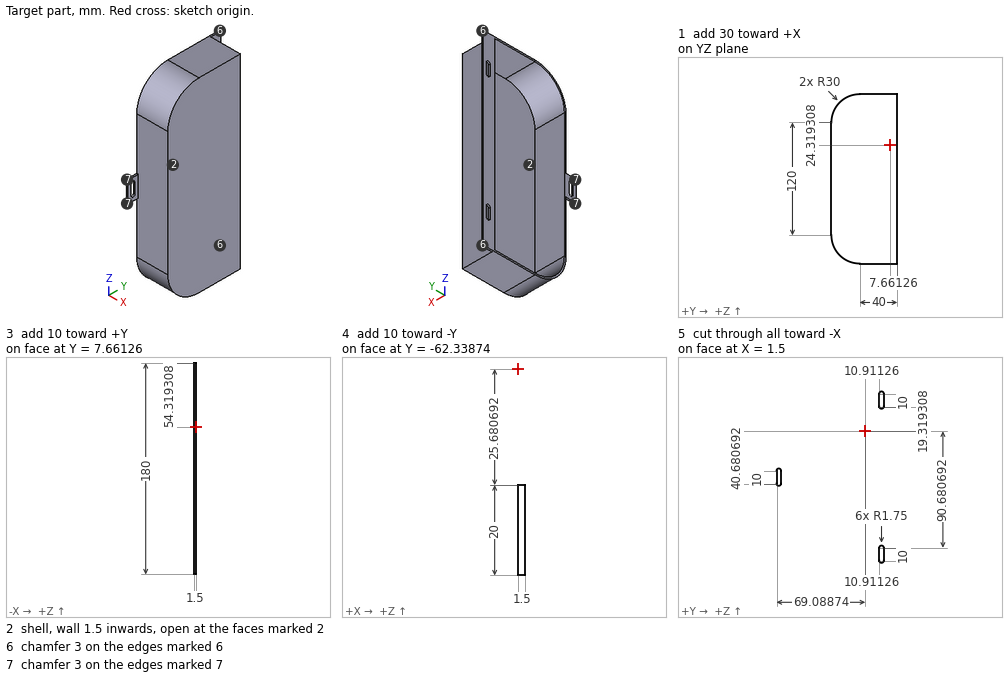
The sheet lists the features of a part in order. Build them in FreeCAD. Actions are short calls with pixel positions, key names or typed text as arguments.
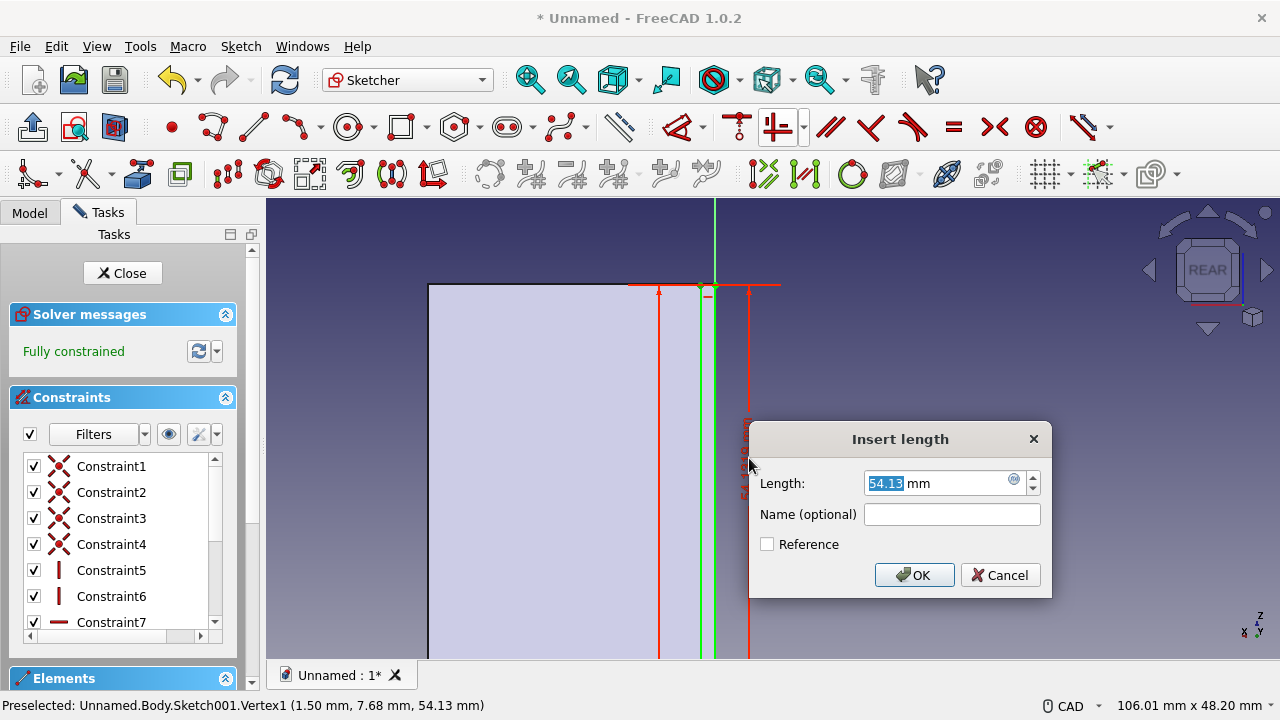
text(54.319308)
key(Return)
key(Escape)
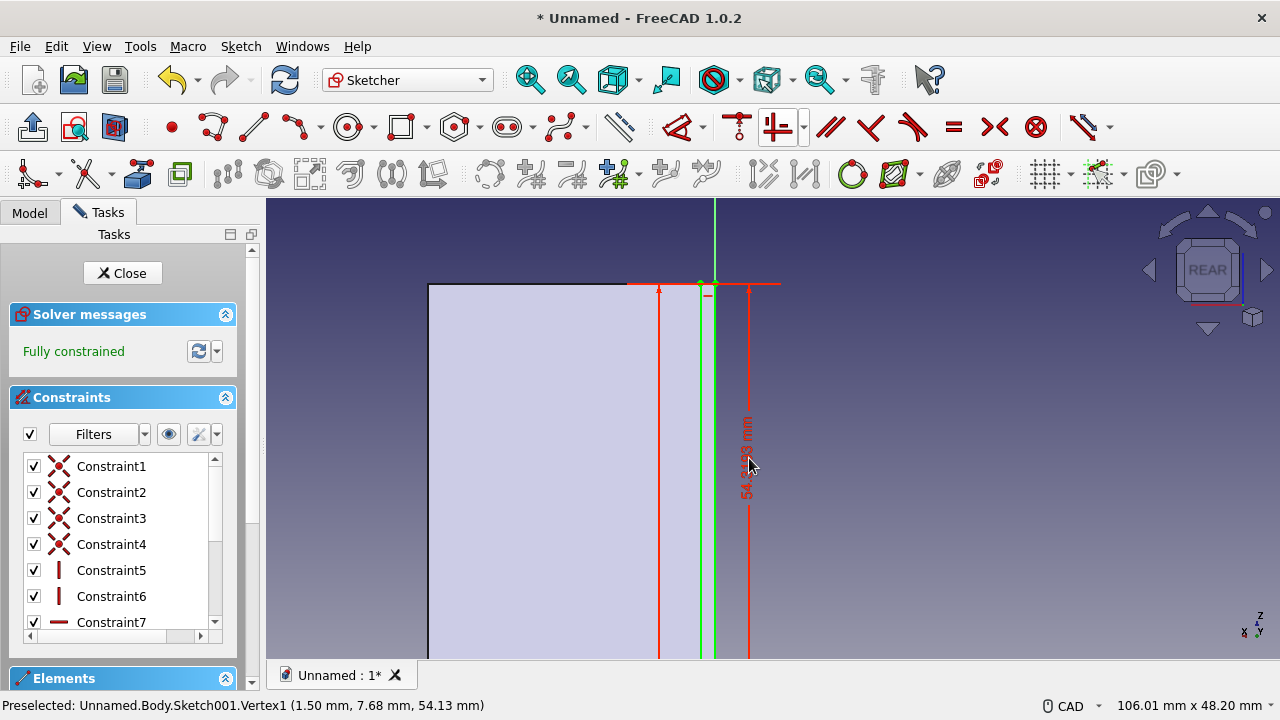
click(123, 273)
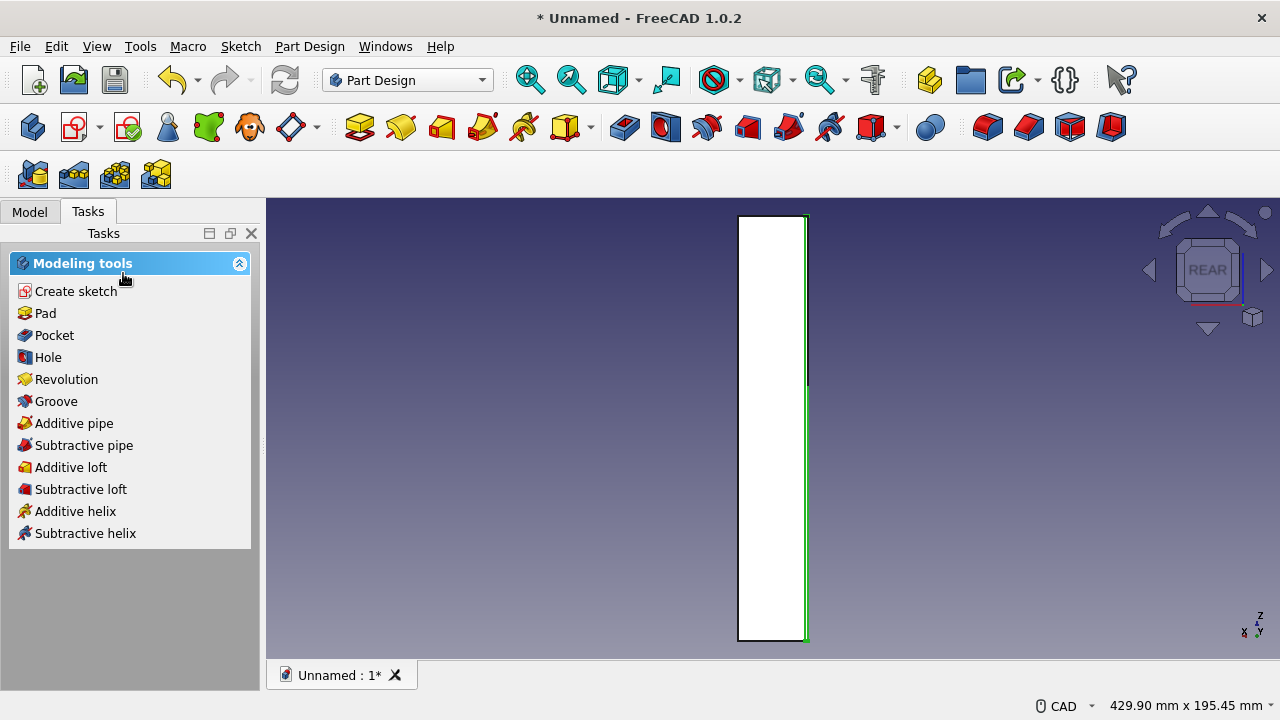
click(360, 128)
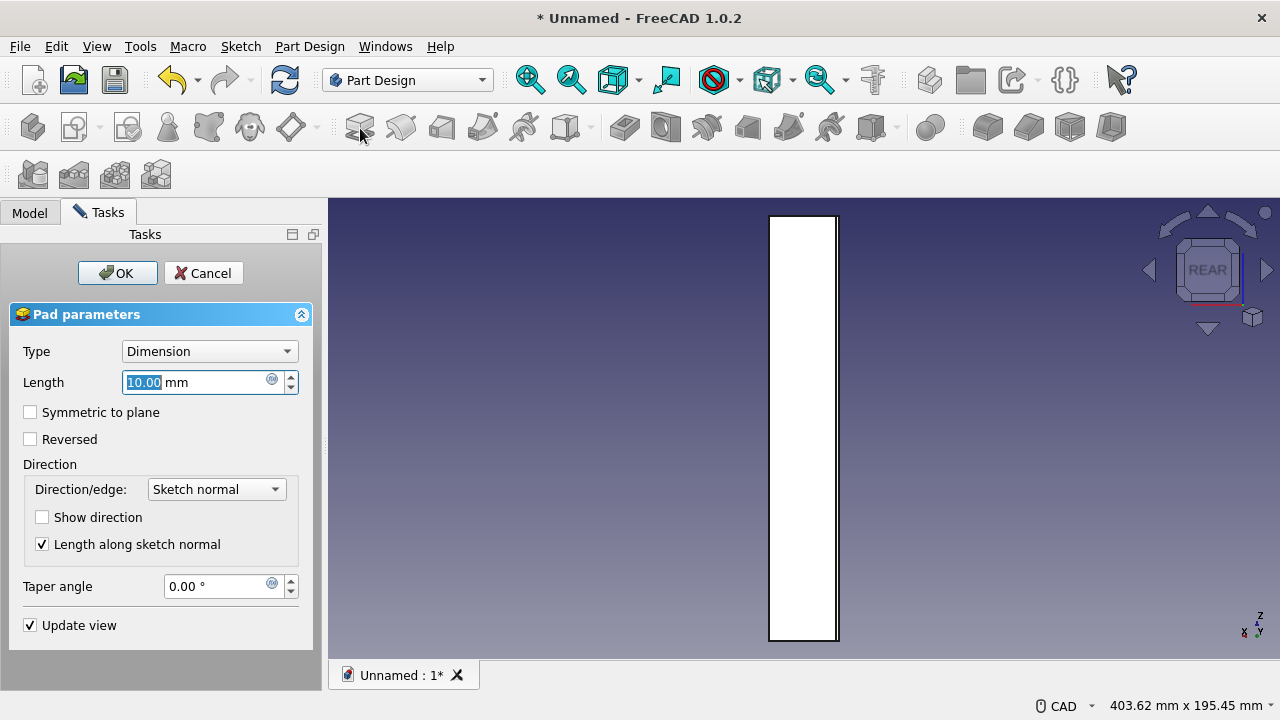
text(10)
key(Tab)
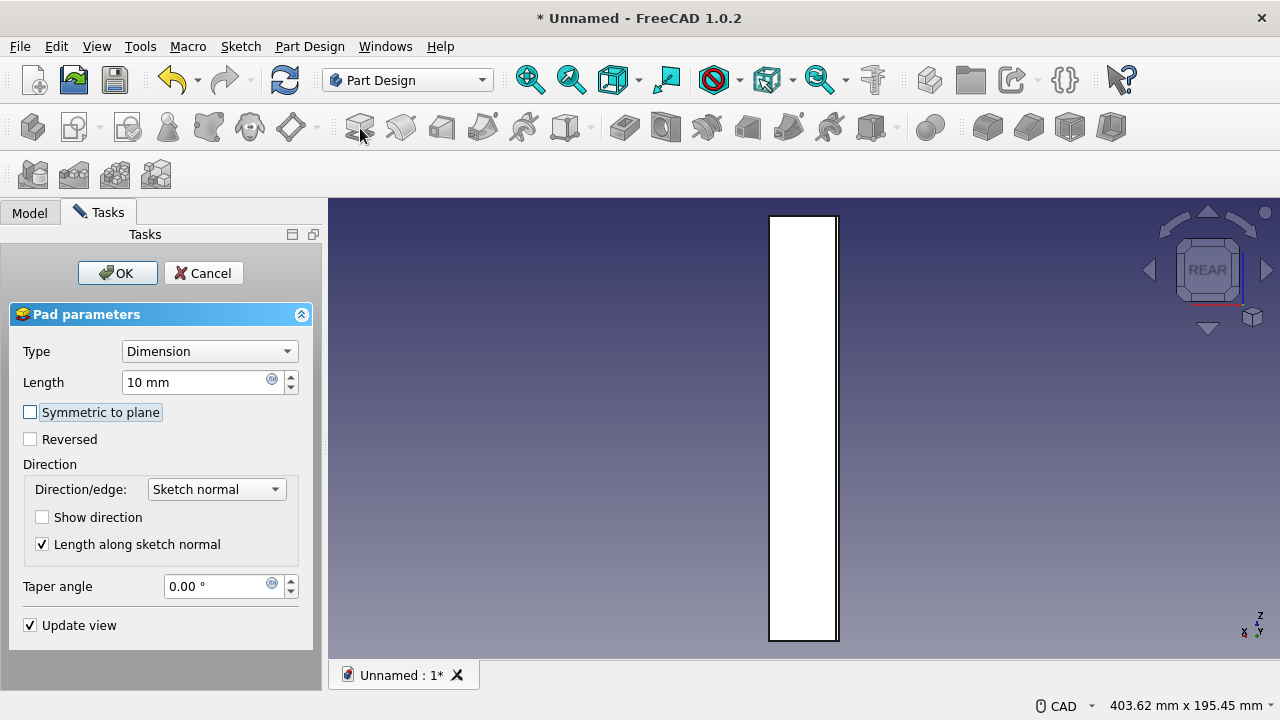
click(118, 273)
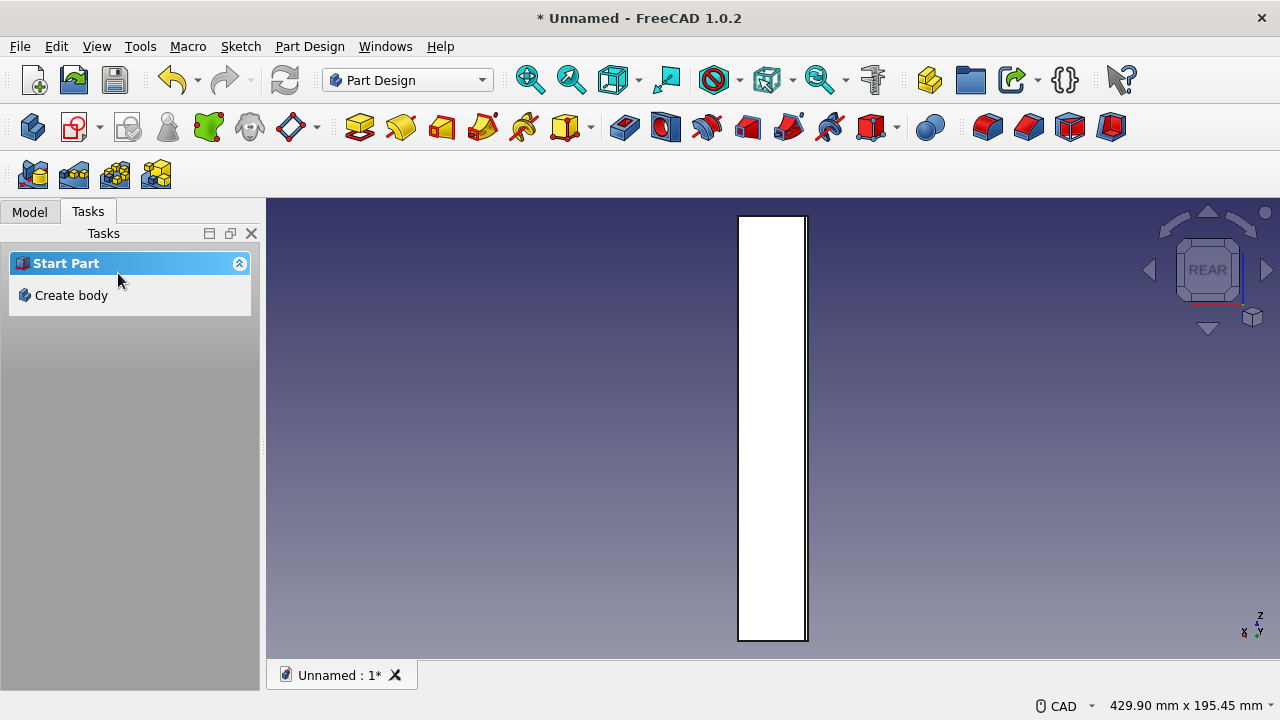
key(0)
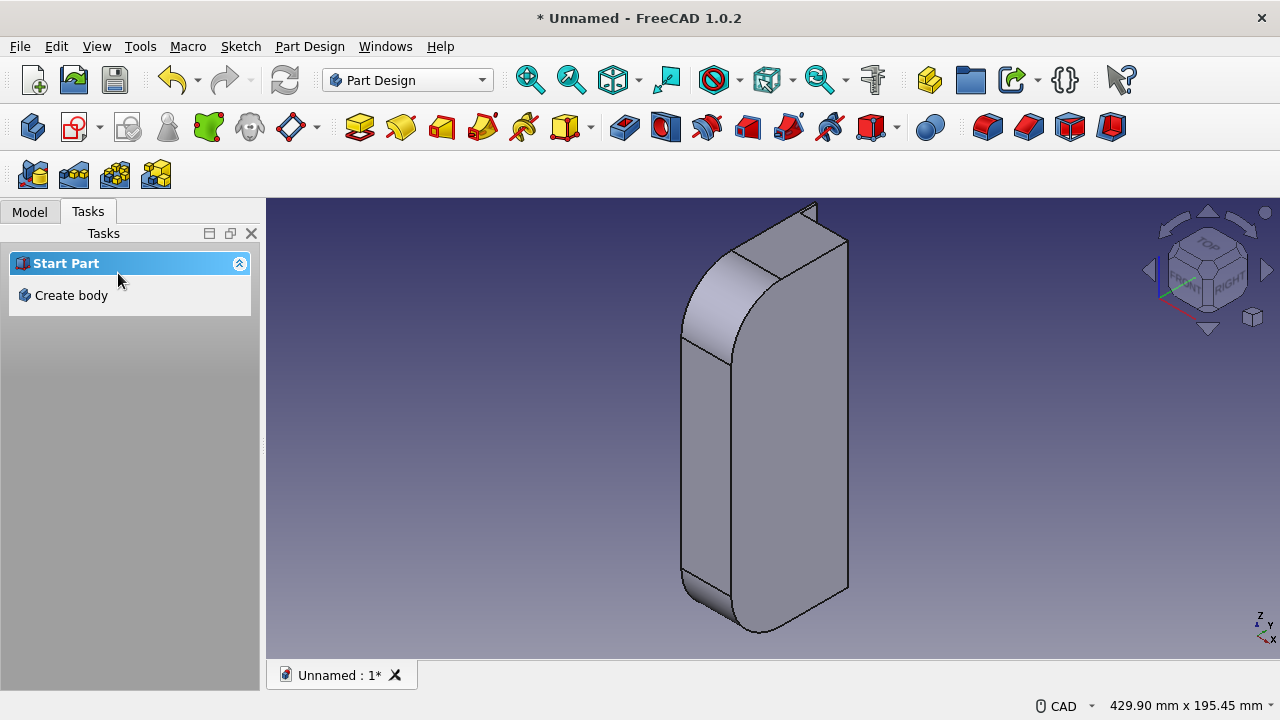
click(706, 532)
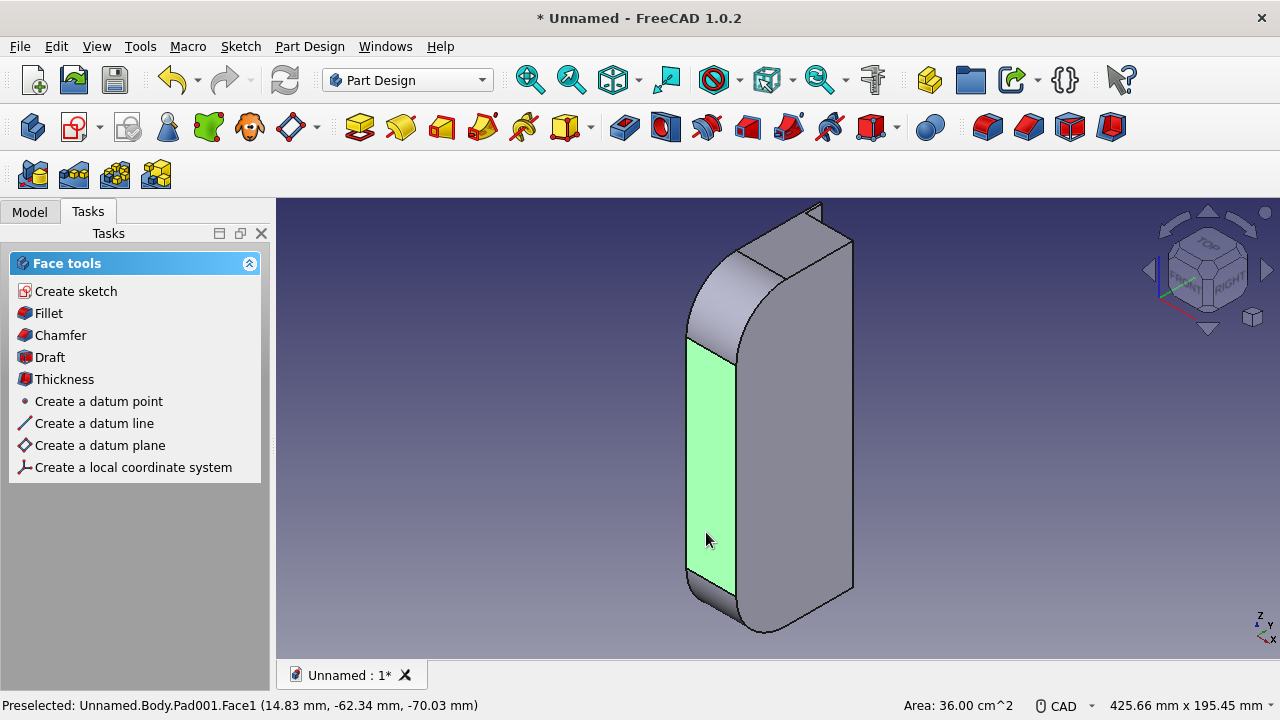
click(74, 128)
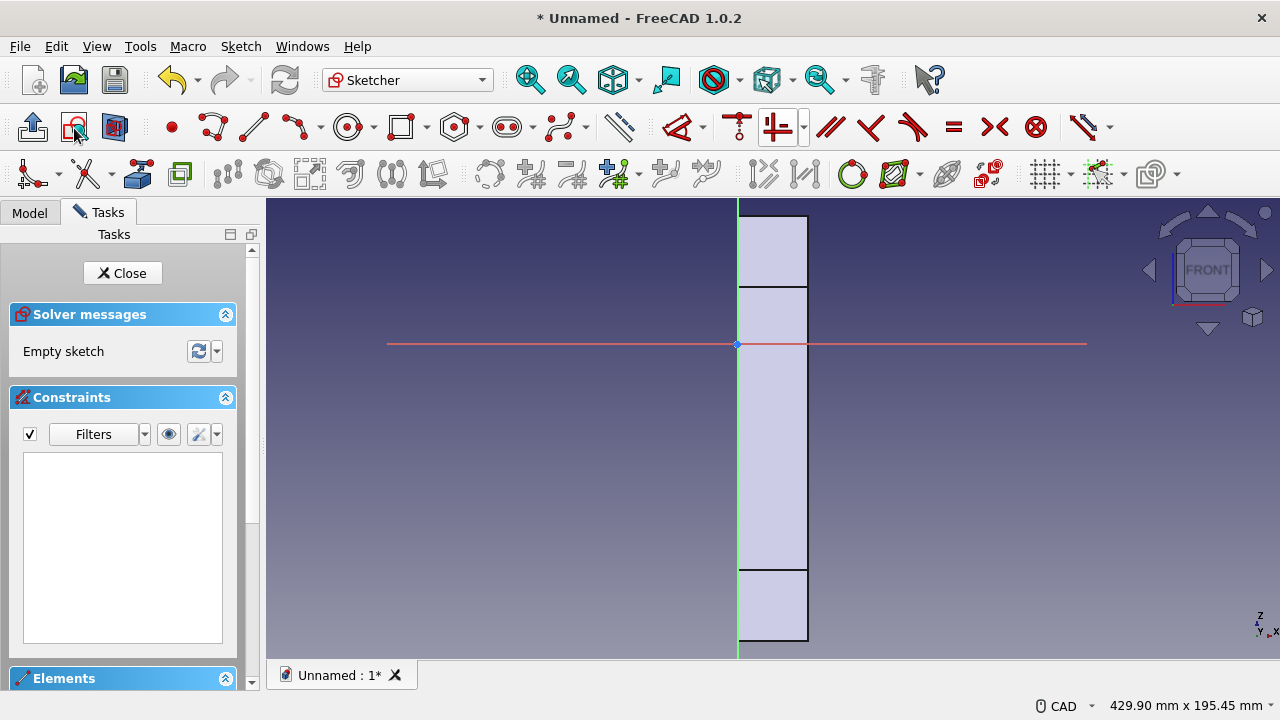
scroll(760, 381, up, 5)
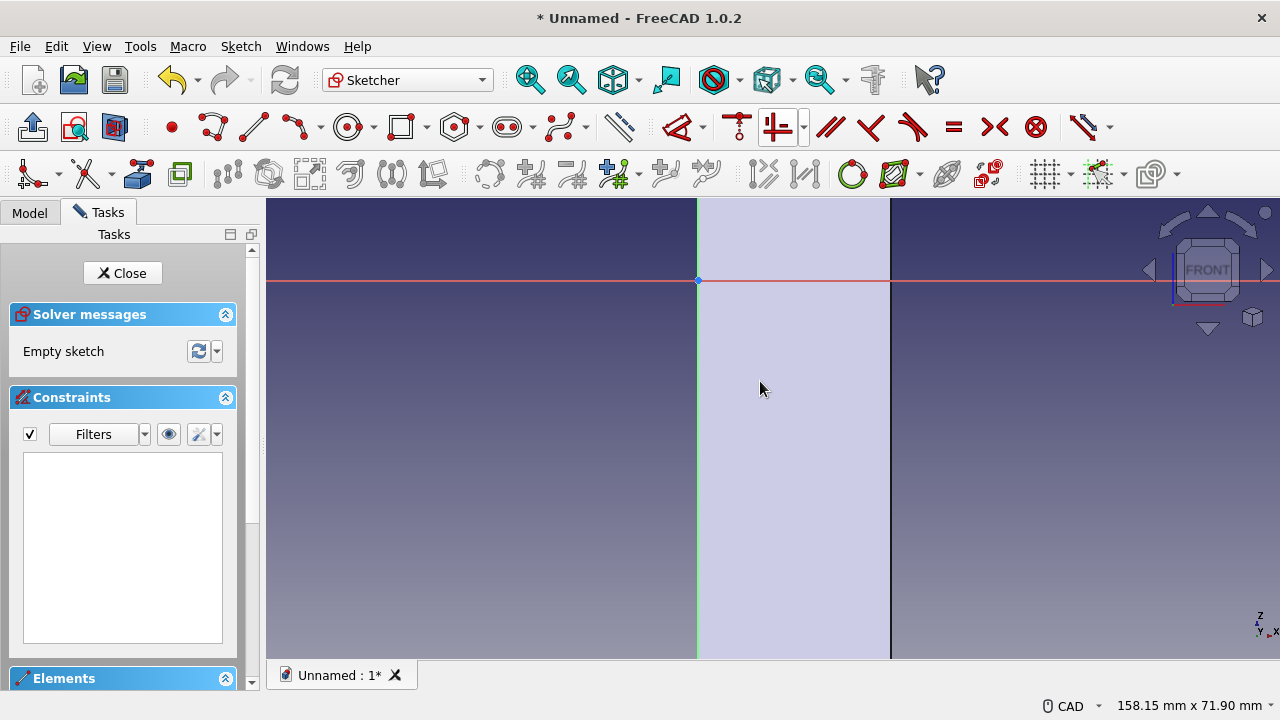
click(400, 128)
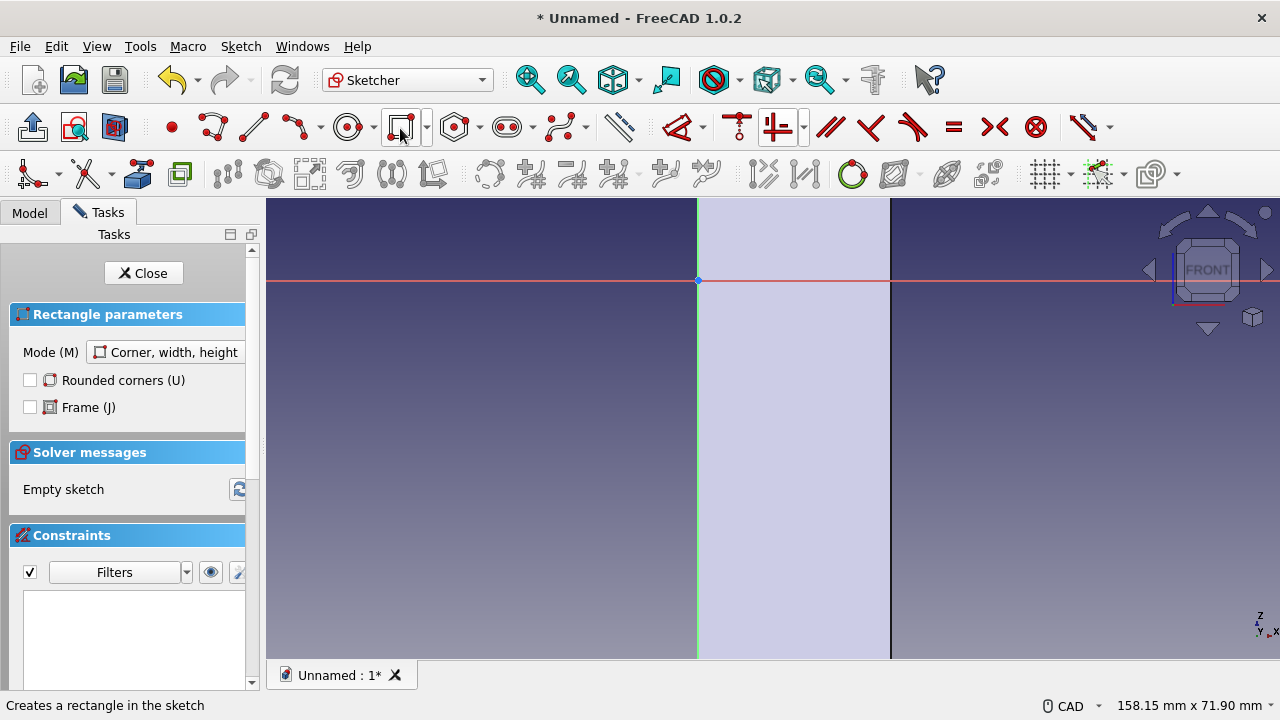
scroll(698, 445, up, 3)